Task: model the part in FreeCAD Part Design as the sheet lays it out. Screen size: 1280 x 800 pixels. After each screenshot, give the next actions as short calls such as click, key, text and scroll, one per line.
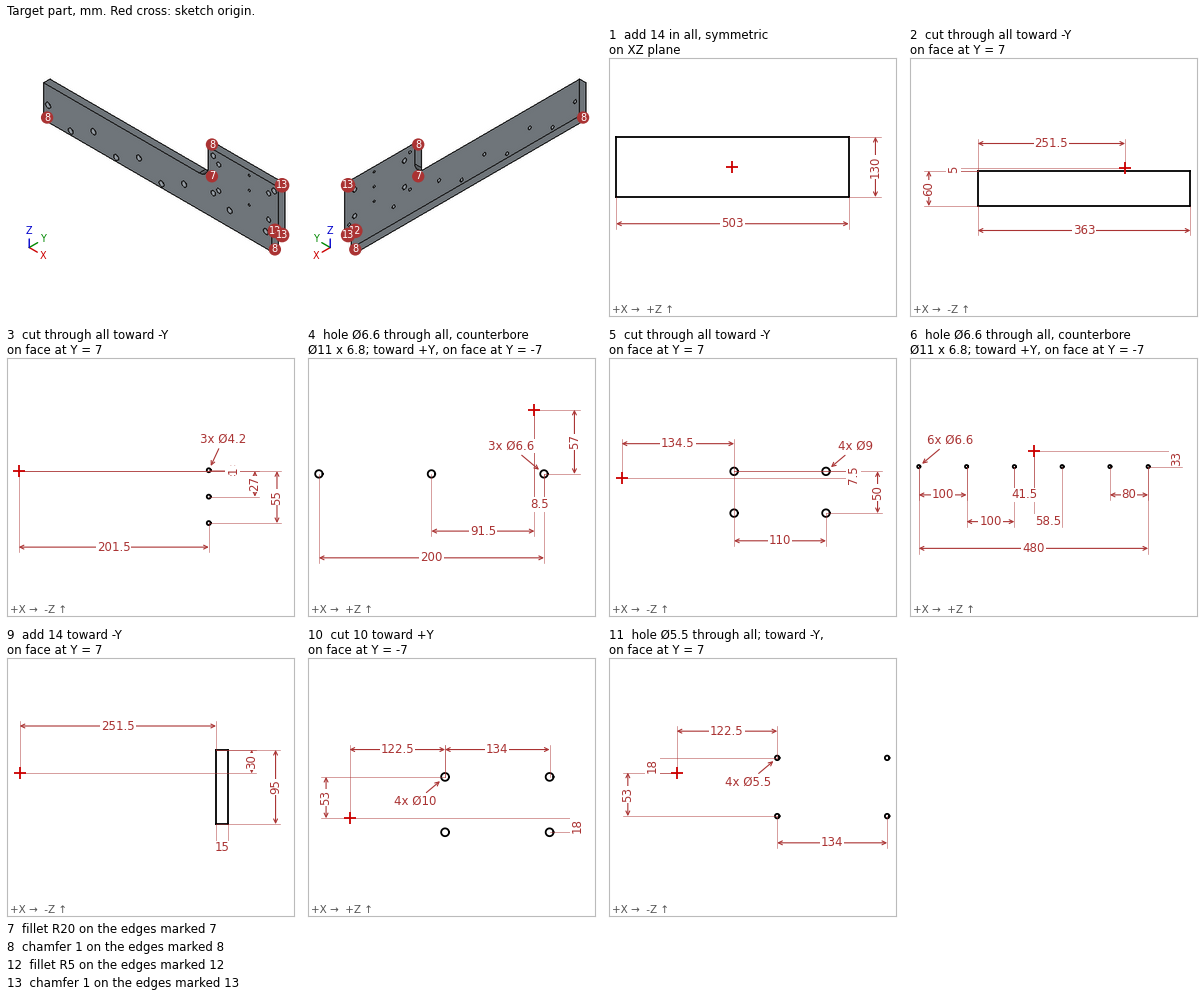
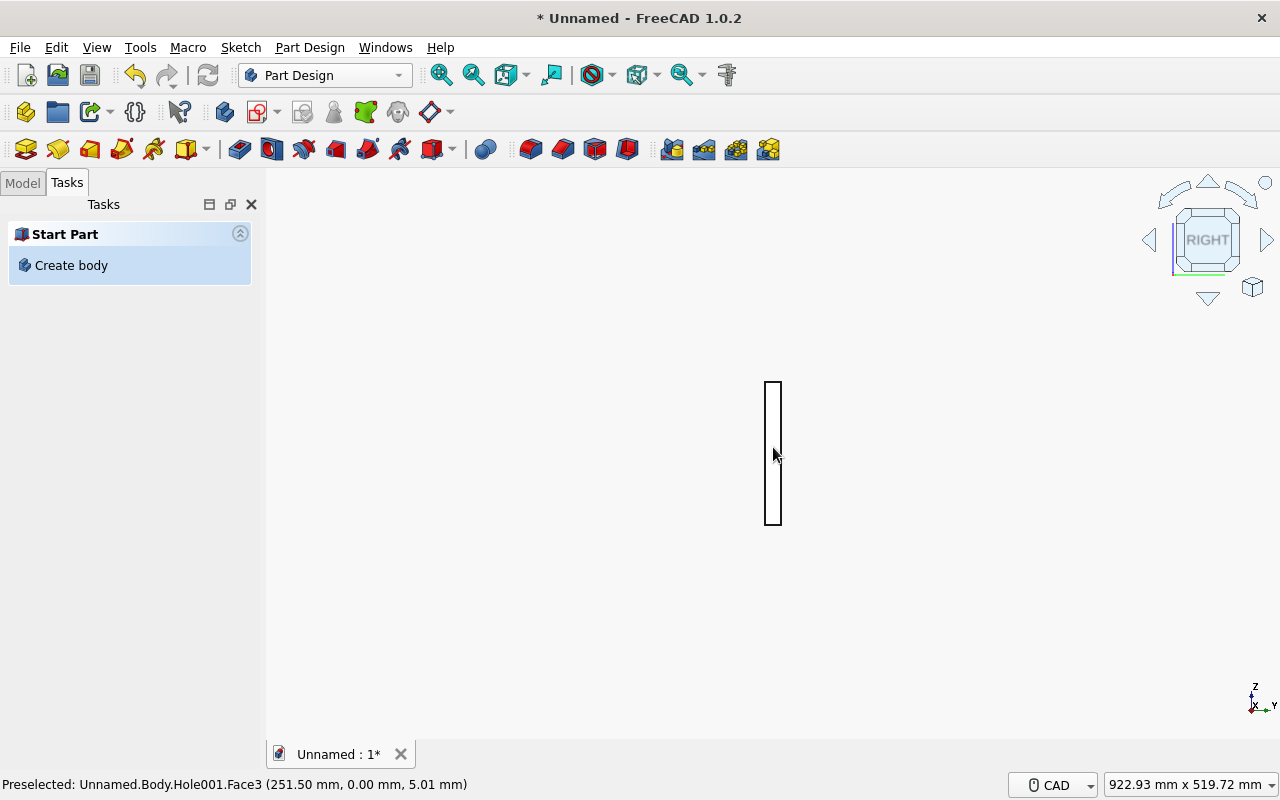
key(5)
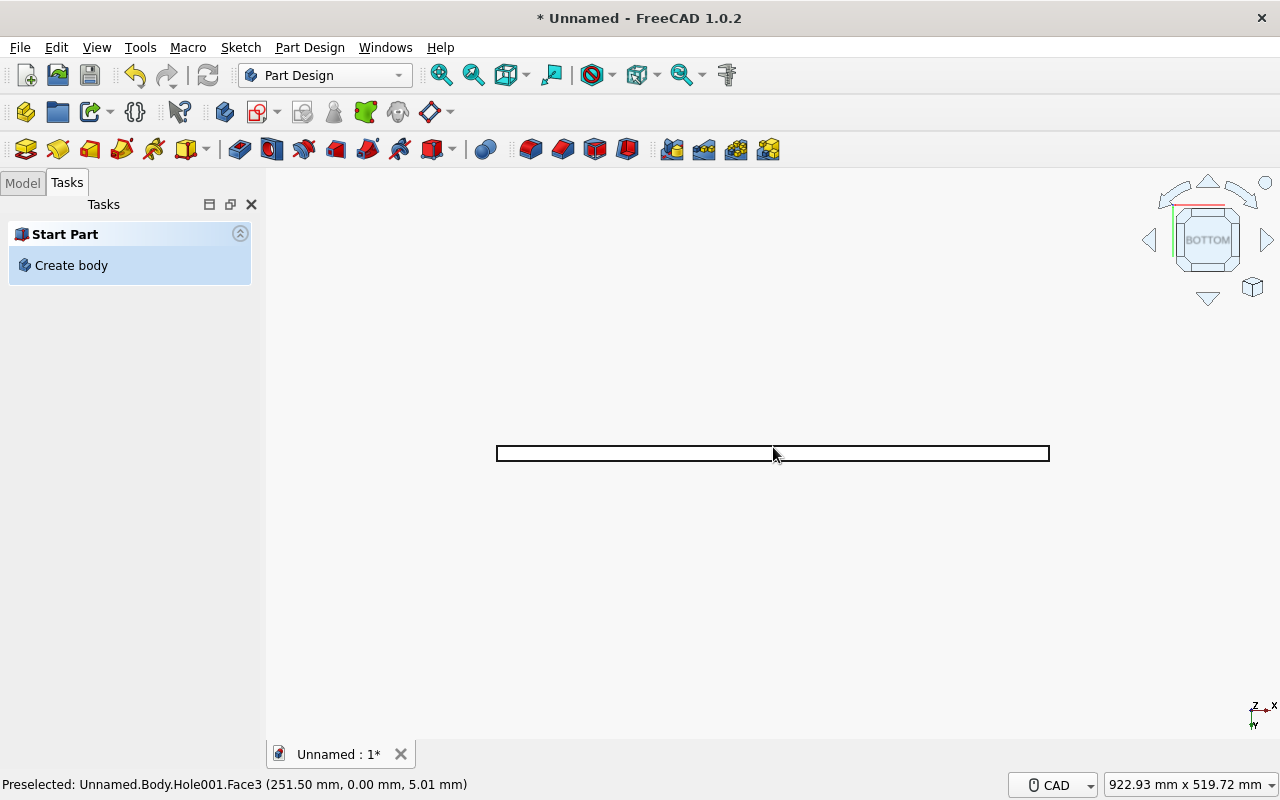
scroll(896, 452, up, 5)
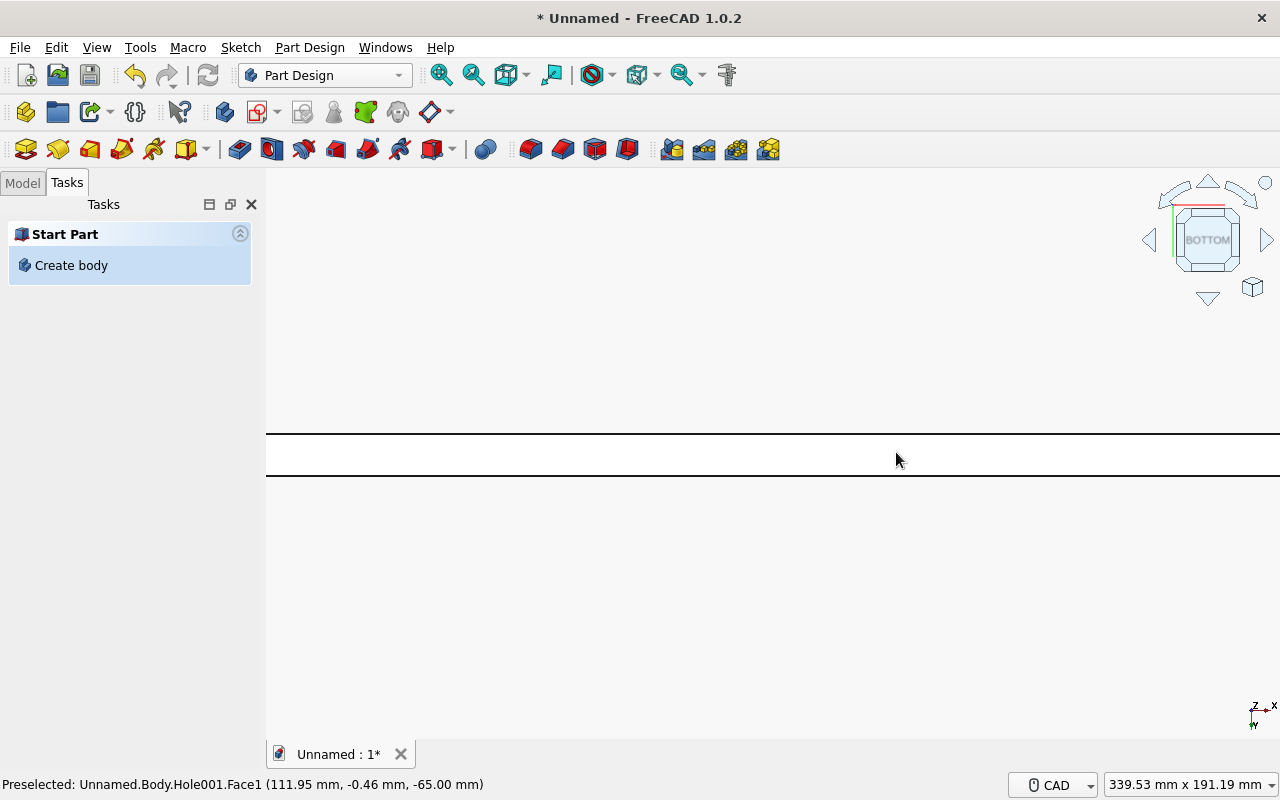
key(v)
key(f)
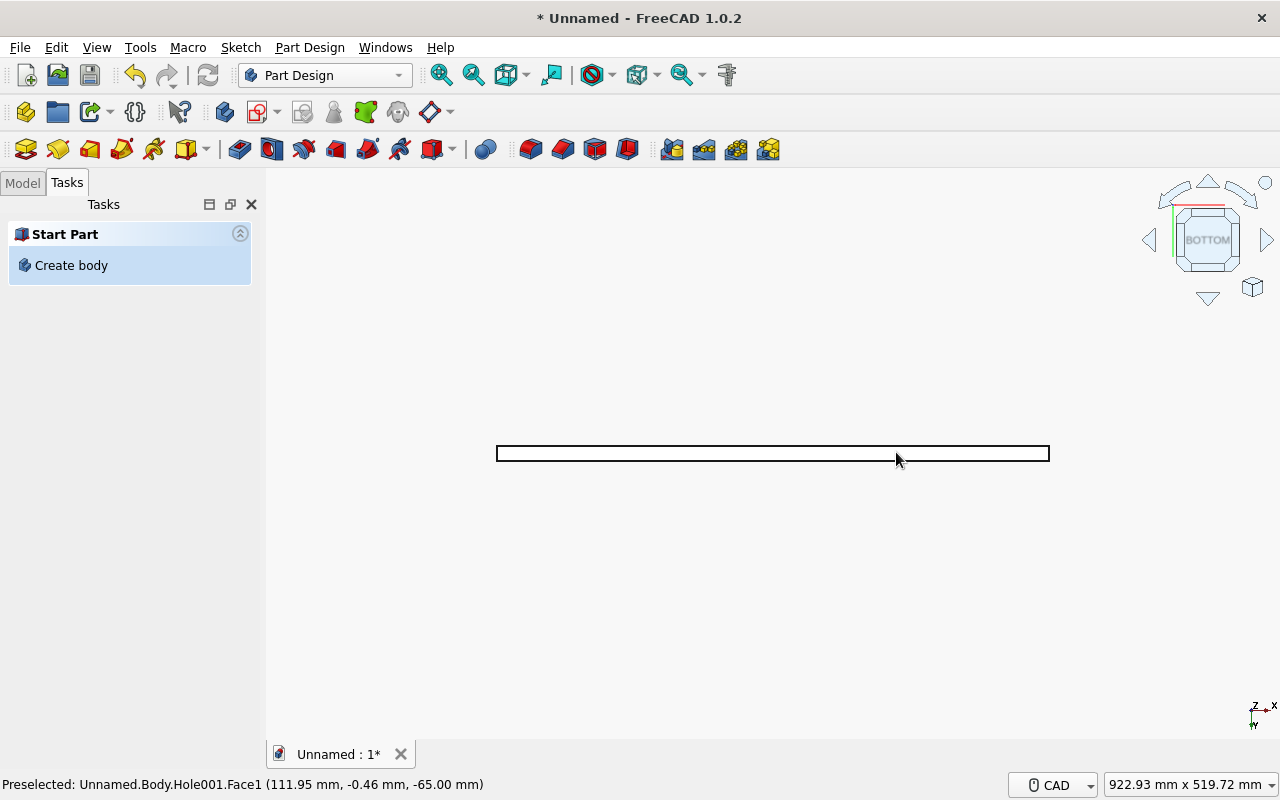
key(4)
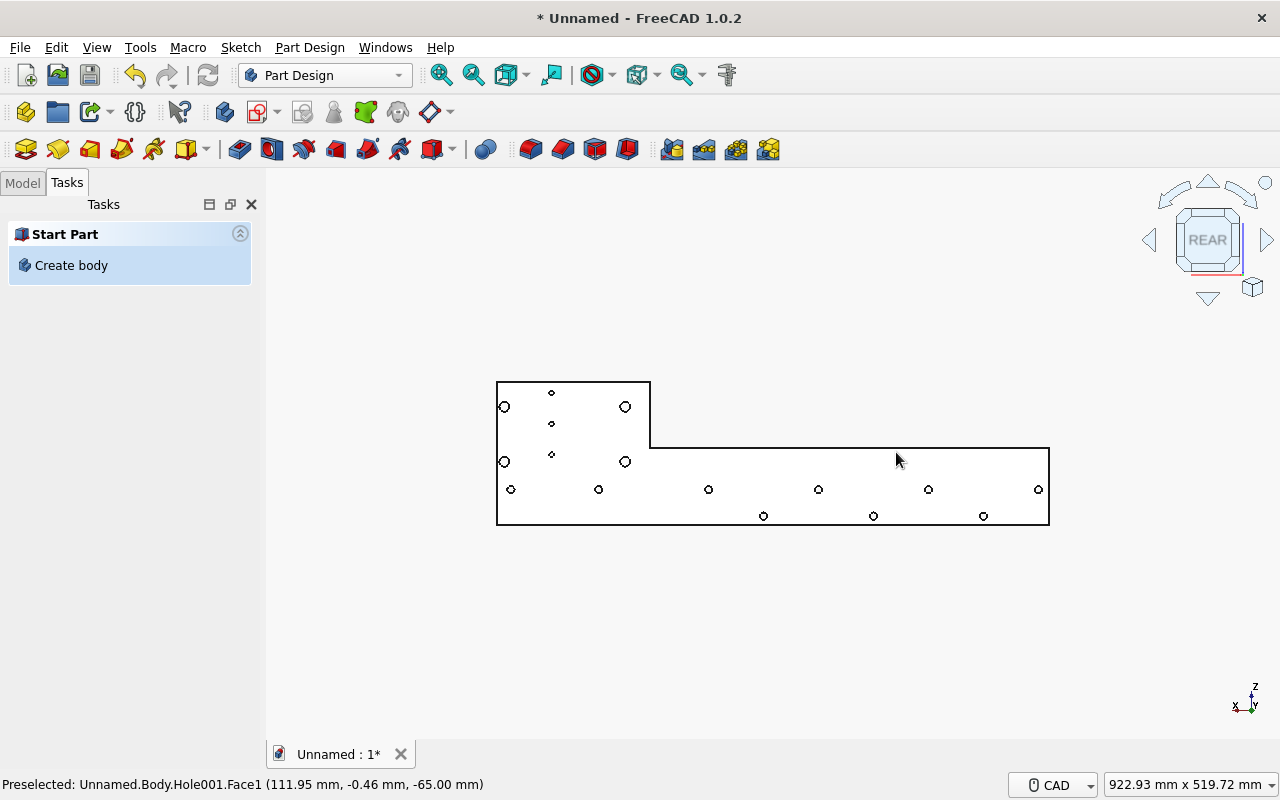
scroll(650, 447, up, 5)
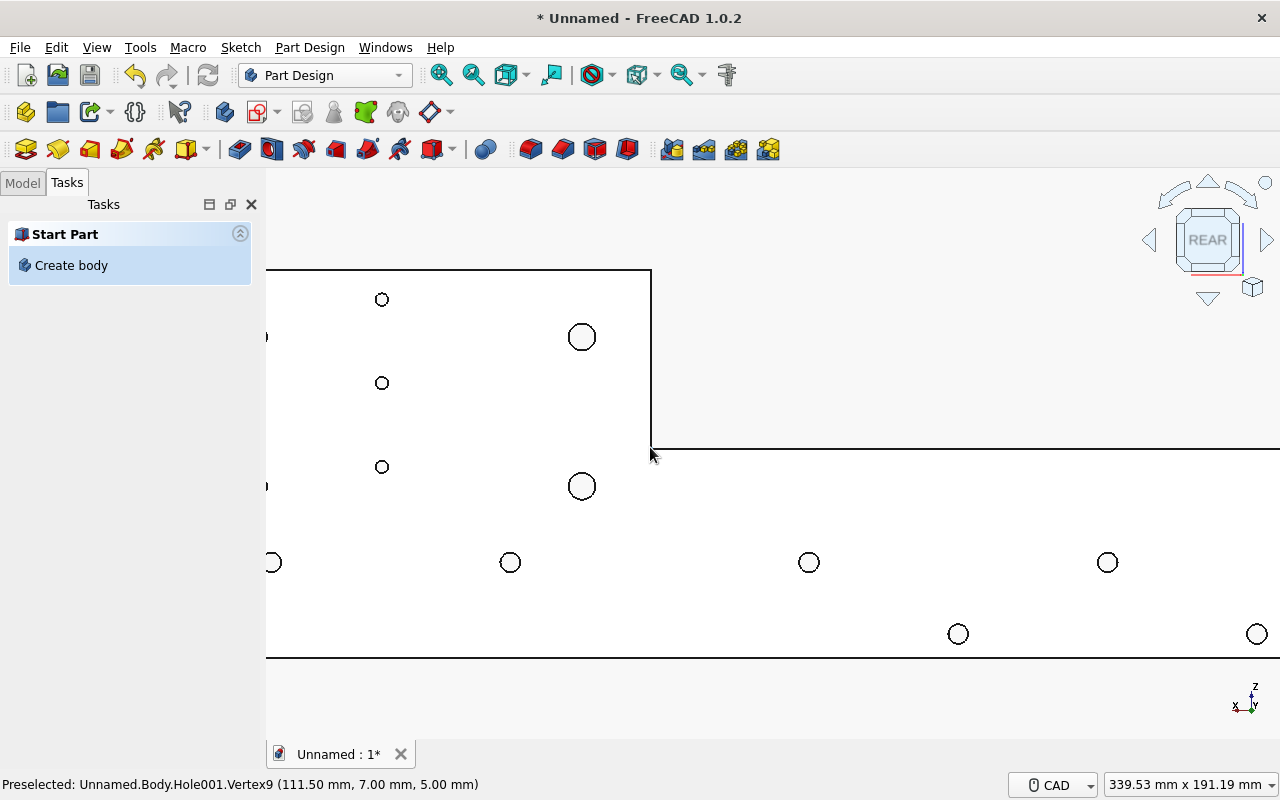
key(v)
key(f)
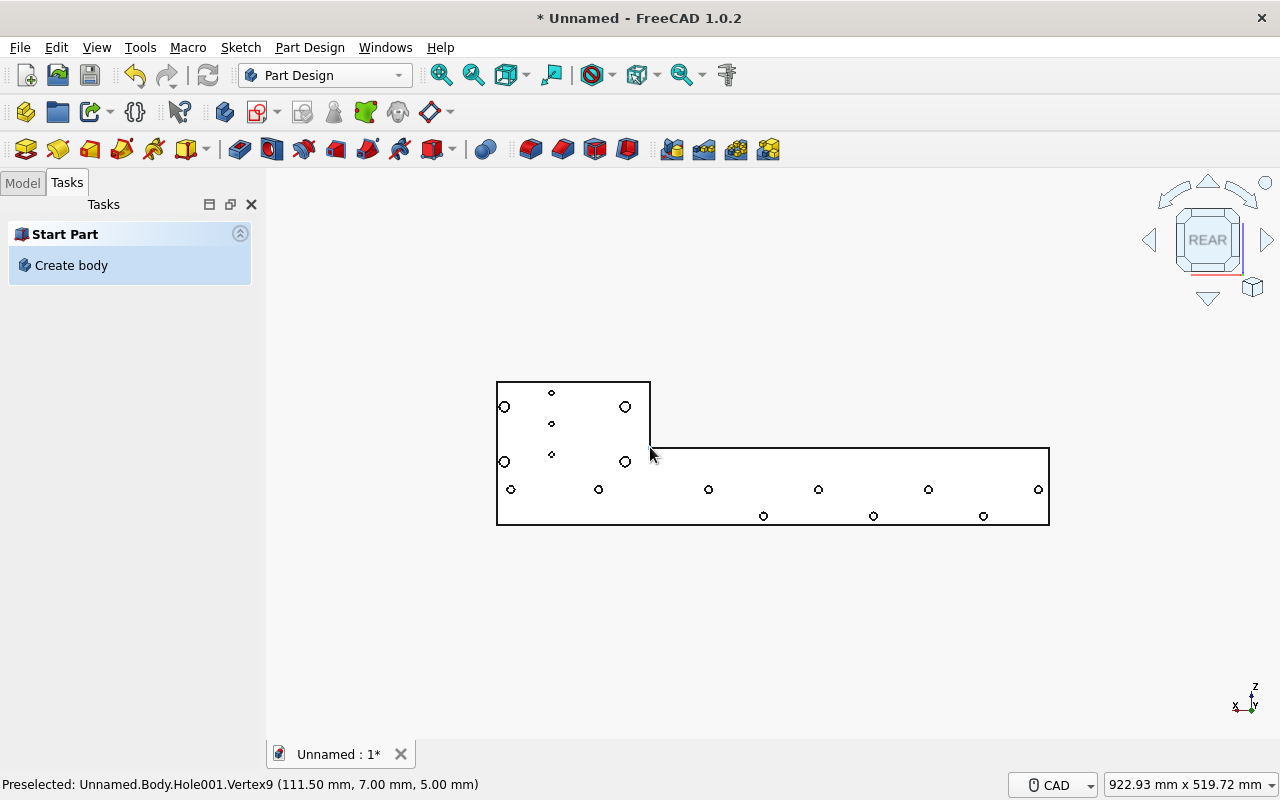
key(6)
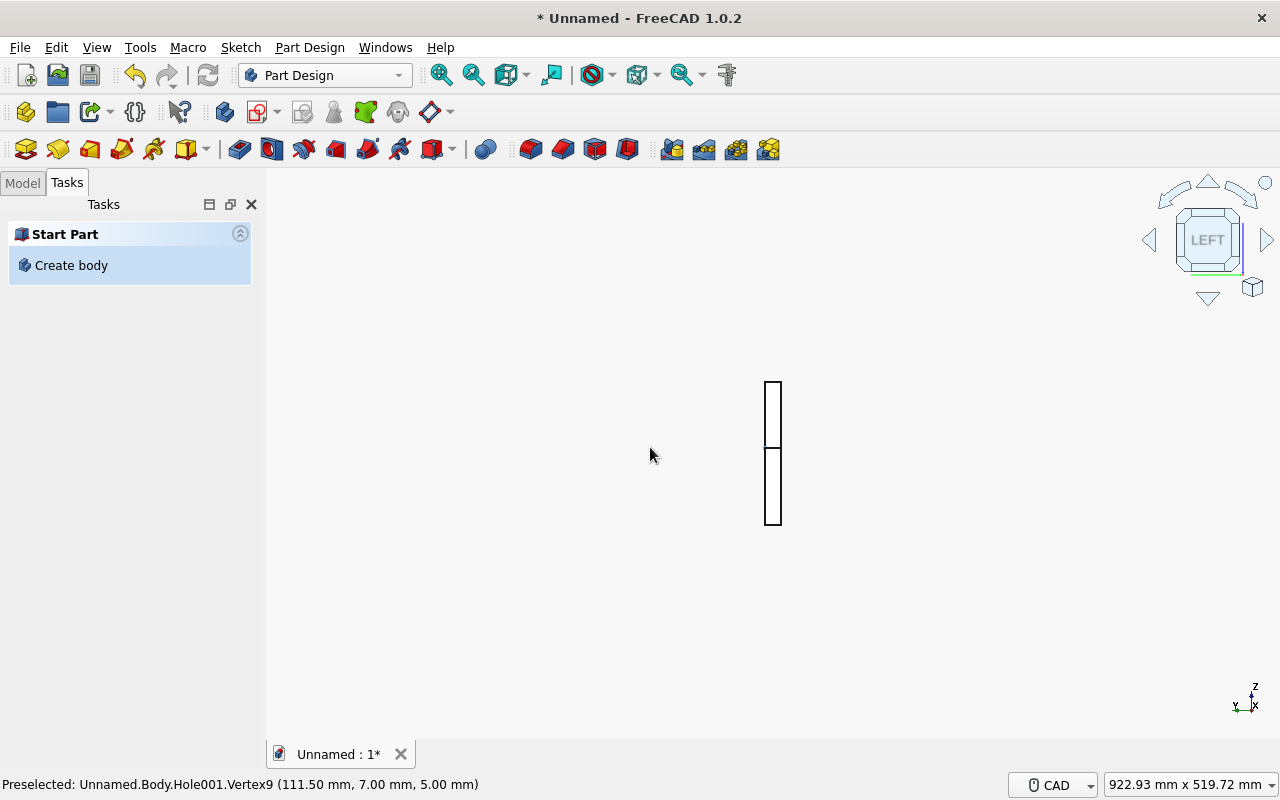
key(v)
key(f)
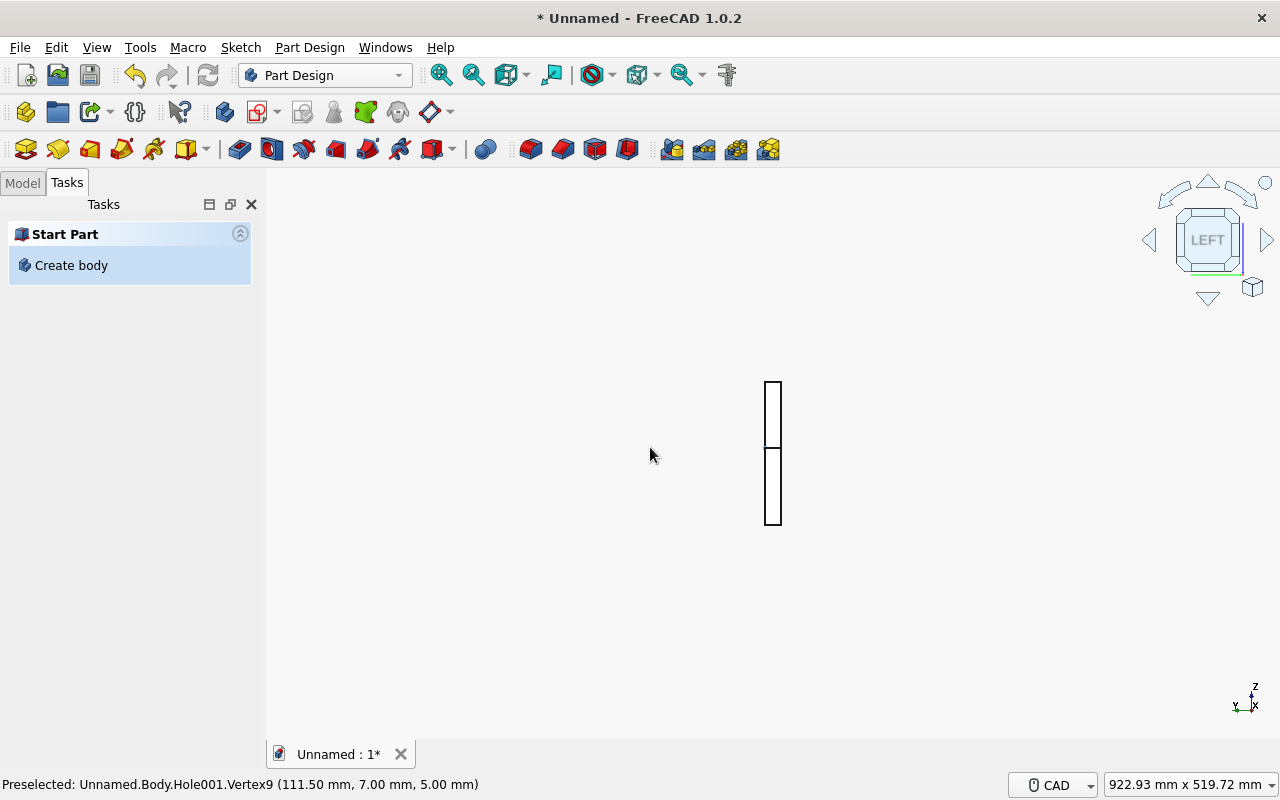
scroll(773, 447, up, 5)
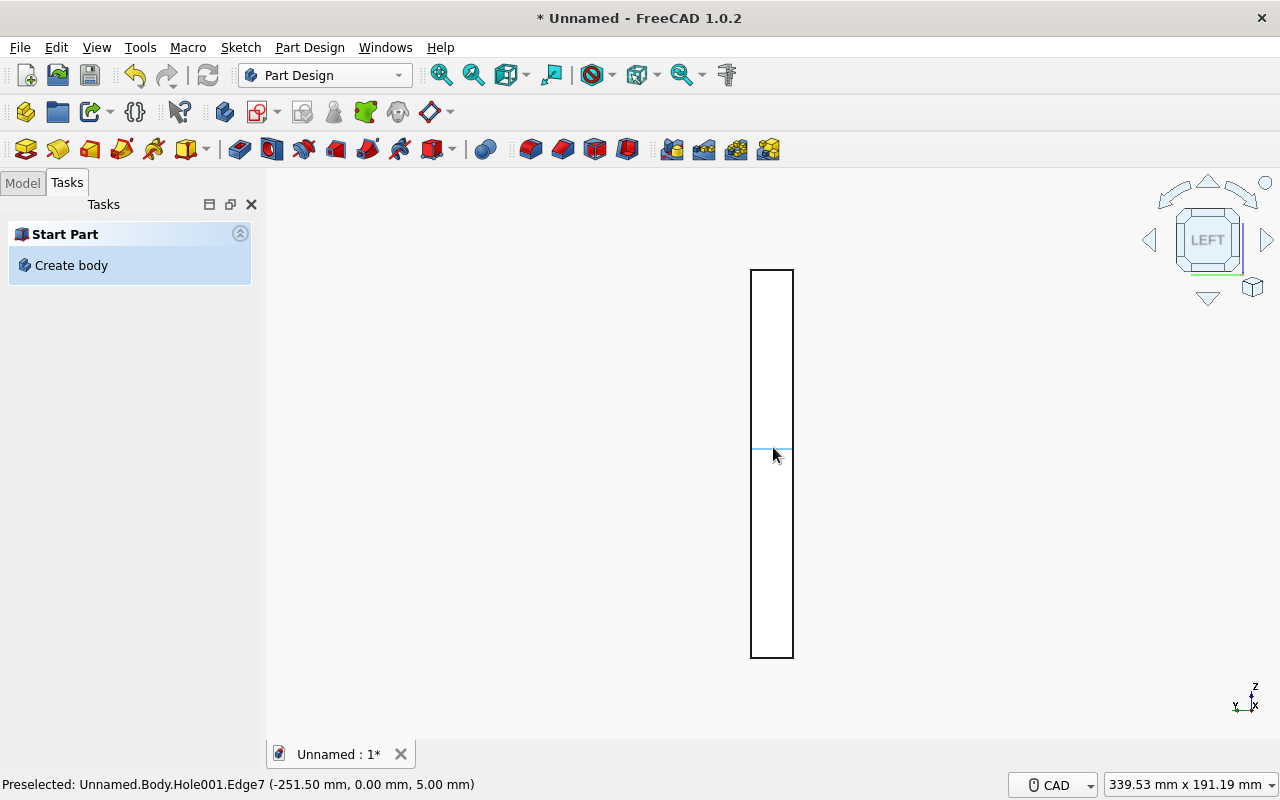
key(v)
key(f)